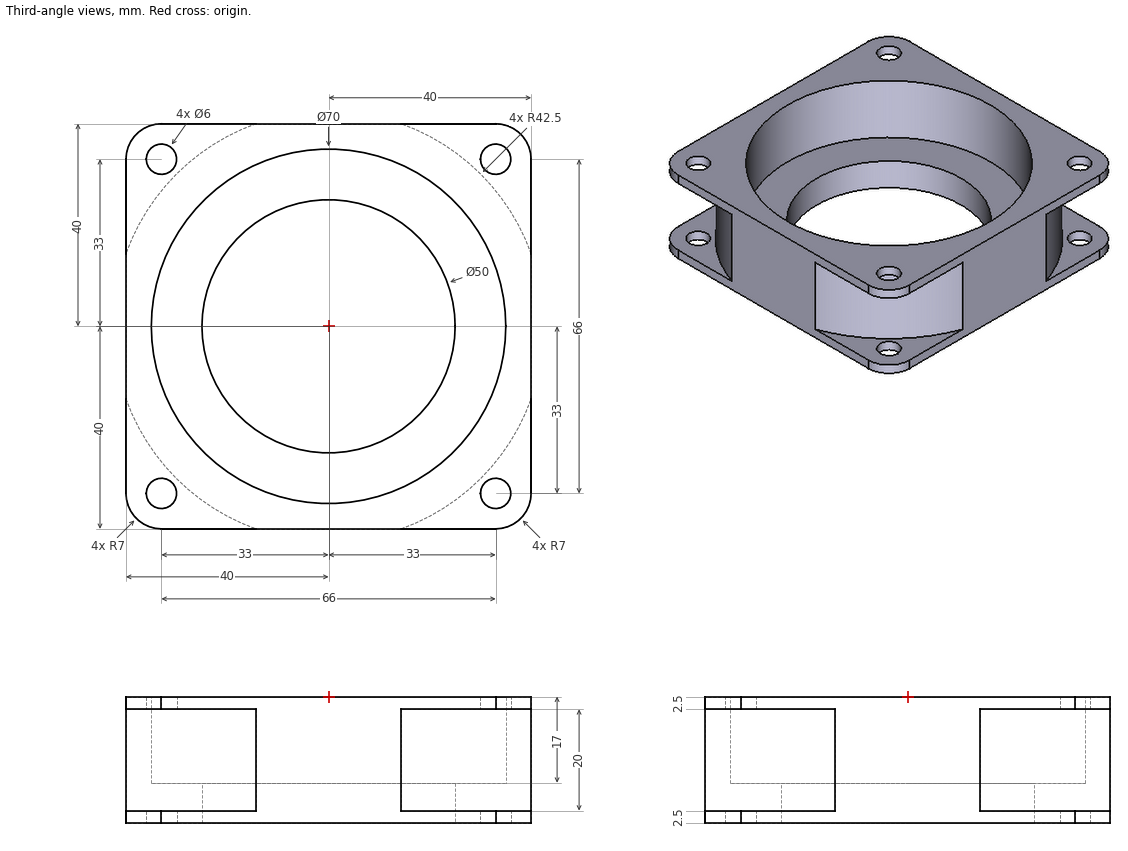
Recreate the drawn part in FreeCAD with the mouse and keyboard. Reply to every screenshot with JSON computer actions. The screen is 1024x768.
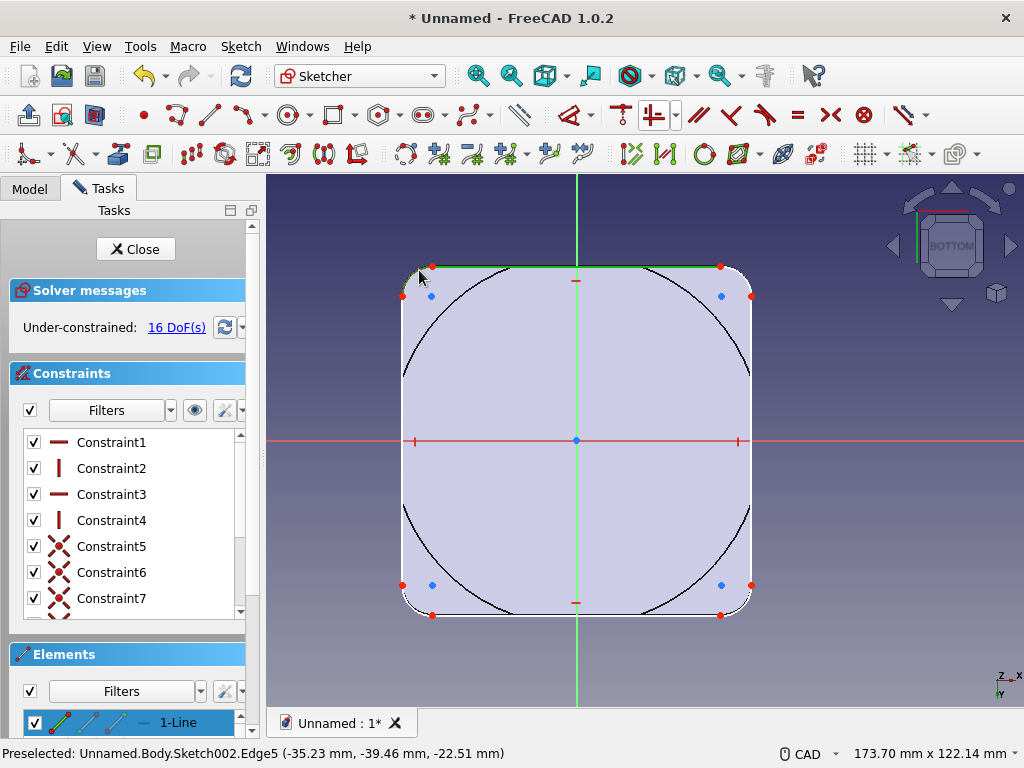
{"action": "left_click", "coordinate": [765, 116]}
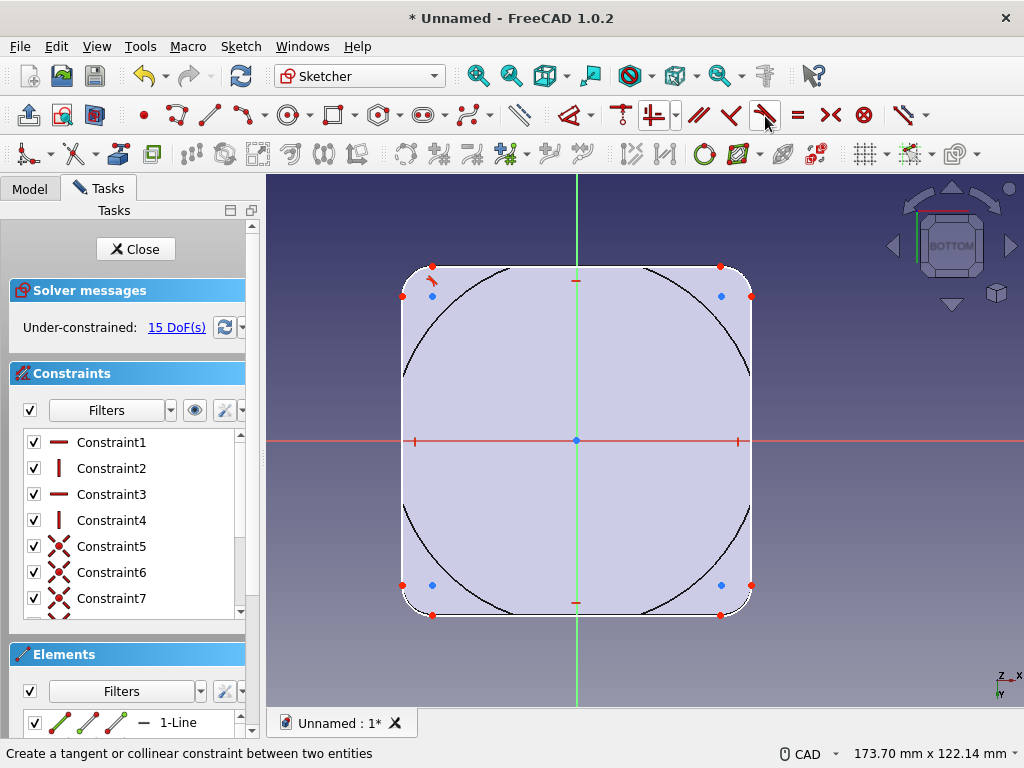
{"action": "left_click", "coordinate": [634, 267]}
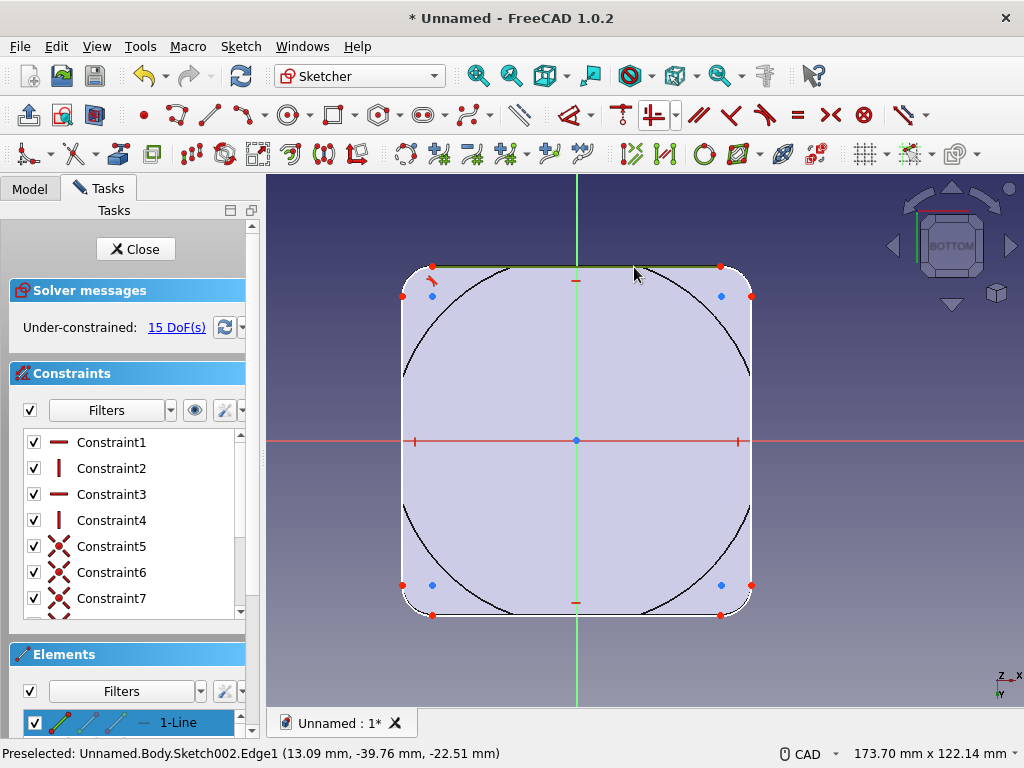
{"action": "left_click", "coordinate": [748, 283]}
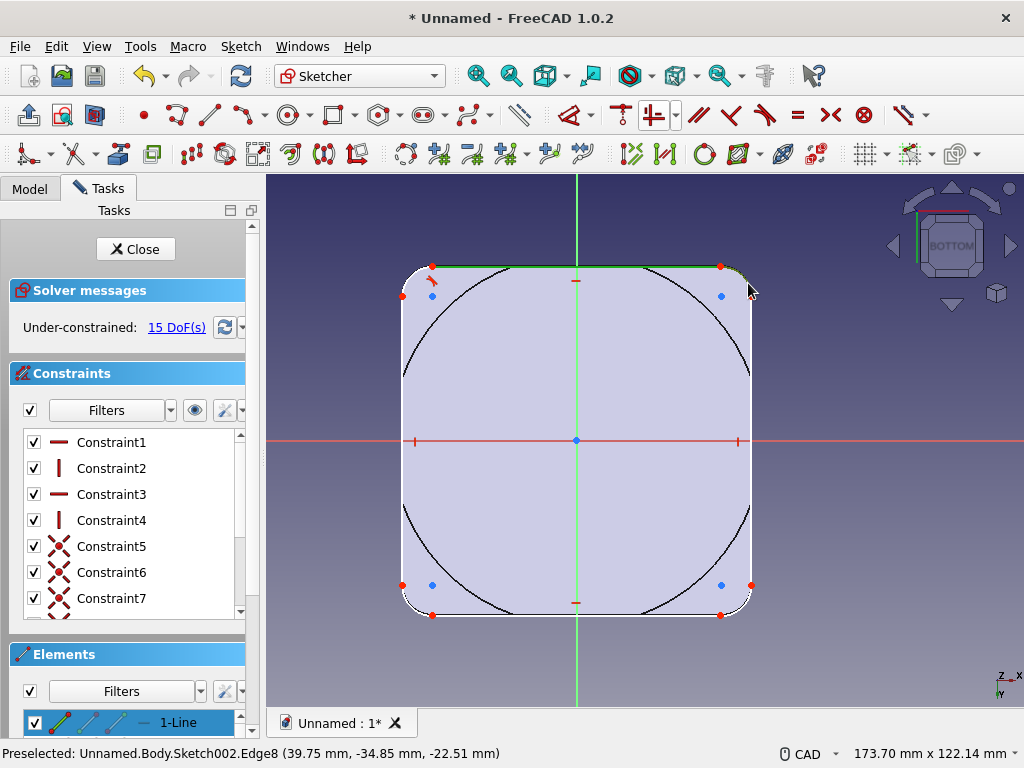
{"action": "left_click", "coordinate": [765, 116]}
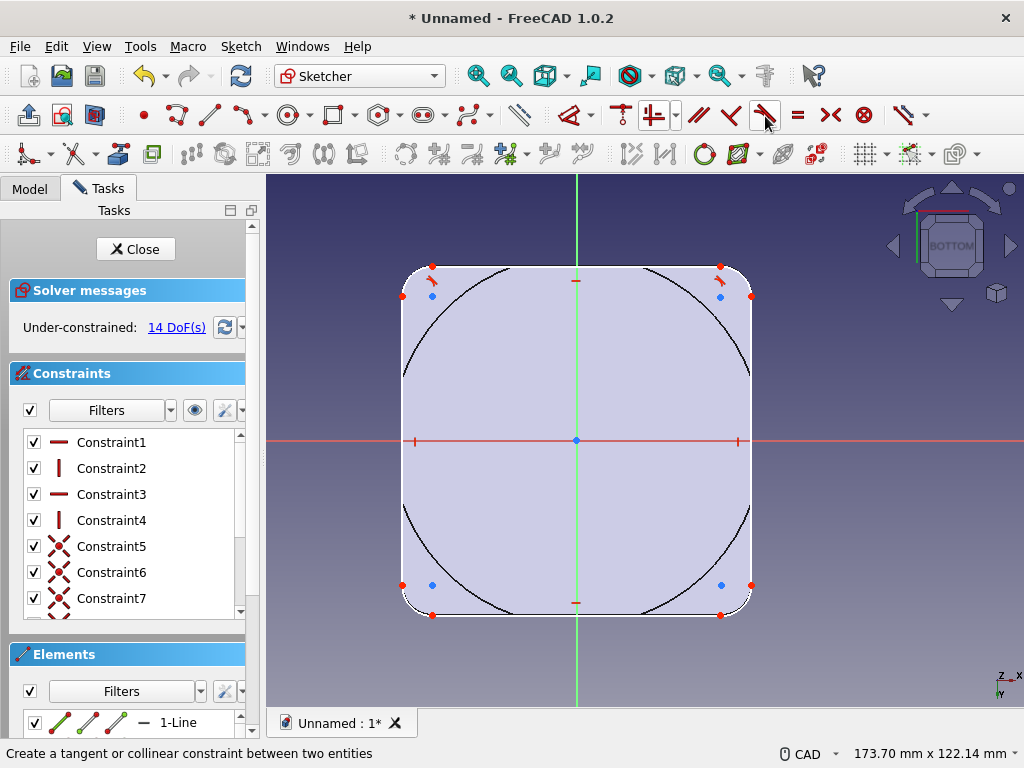
{"action": "left_click", "coordinate": [402, 384]}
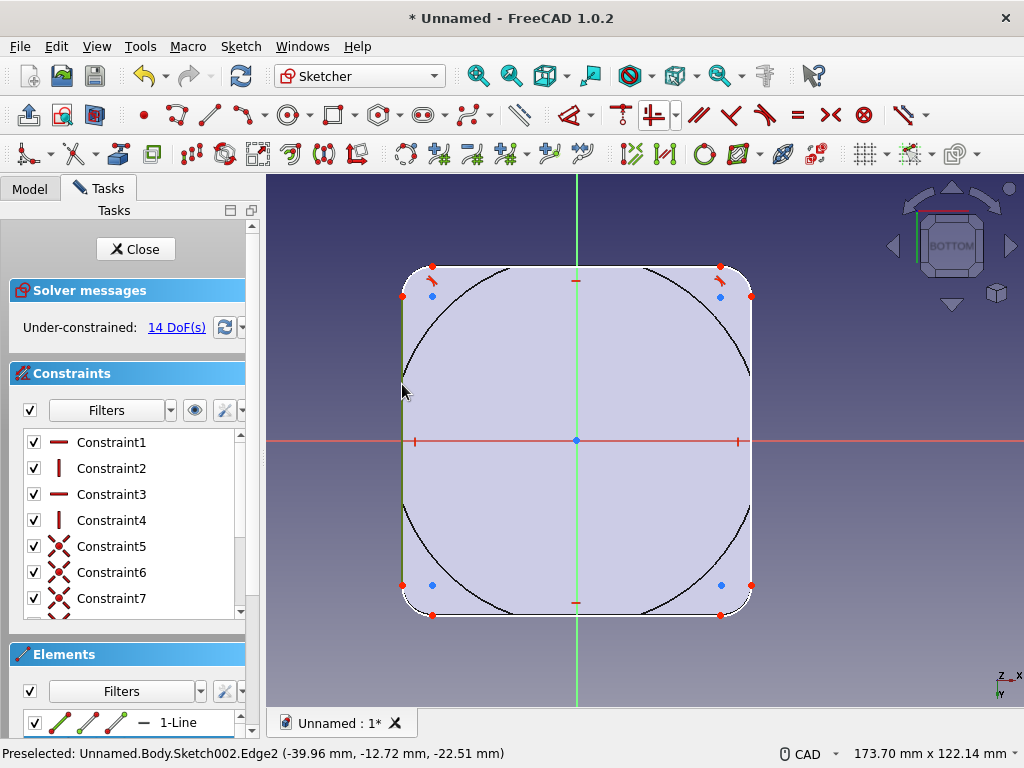
{"action": "left_click", "coordinate": [419, 270]}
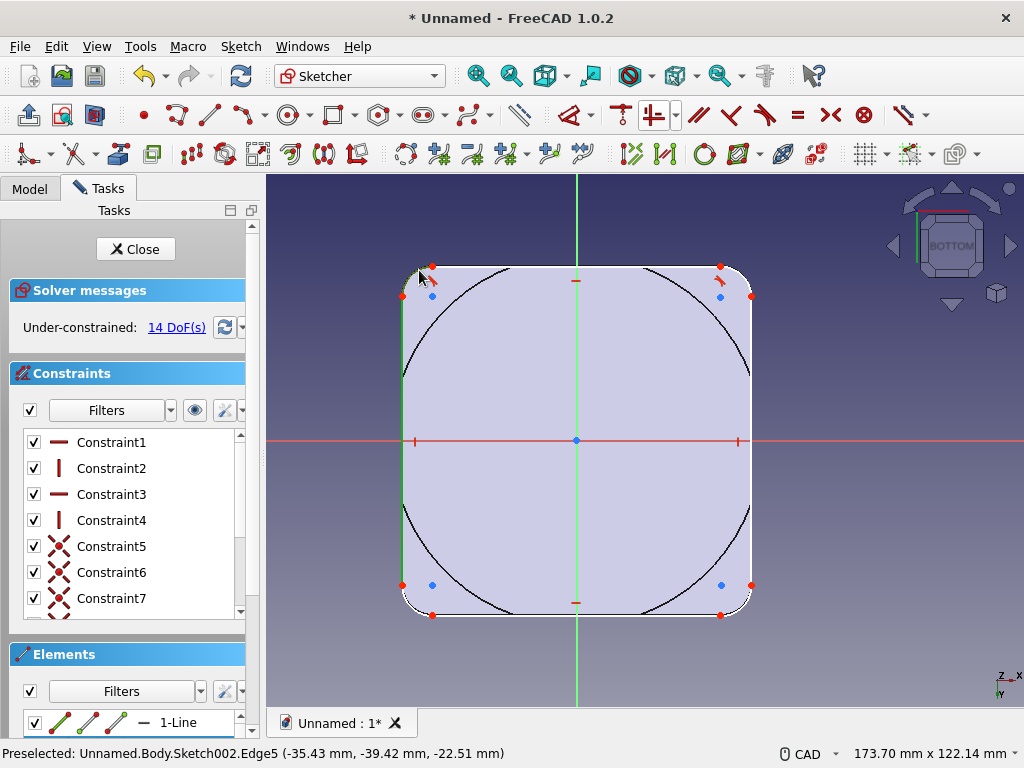
{"action": "left_click", "coordinate": [765, 116]}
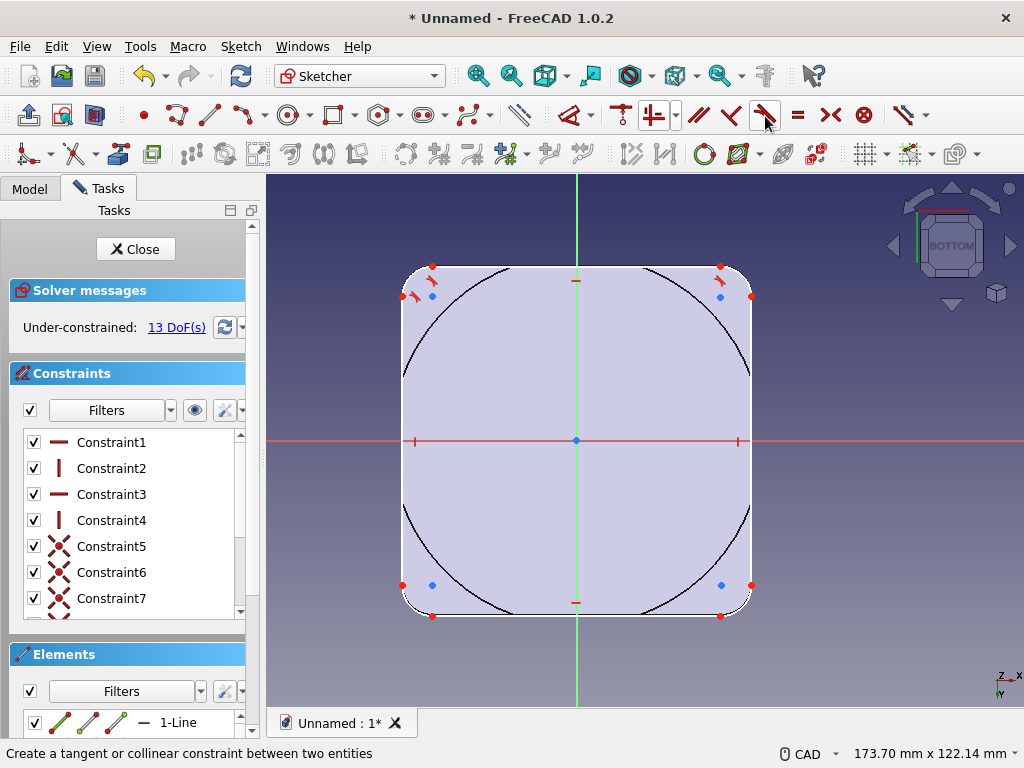
{"action": "left_click", "coordinate": [402, 384]}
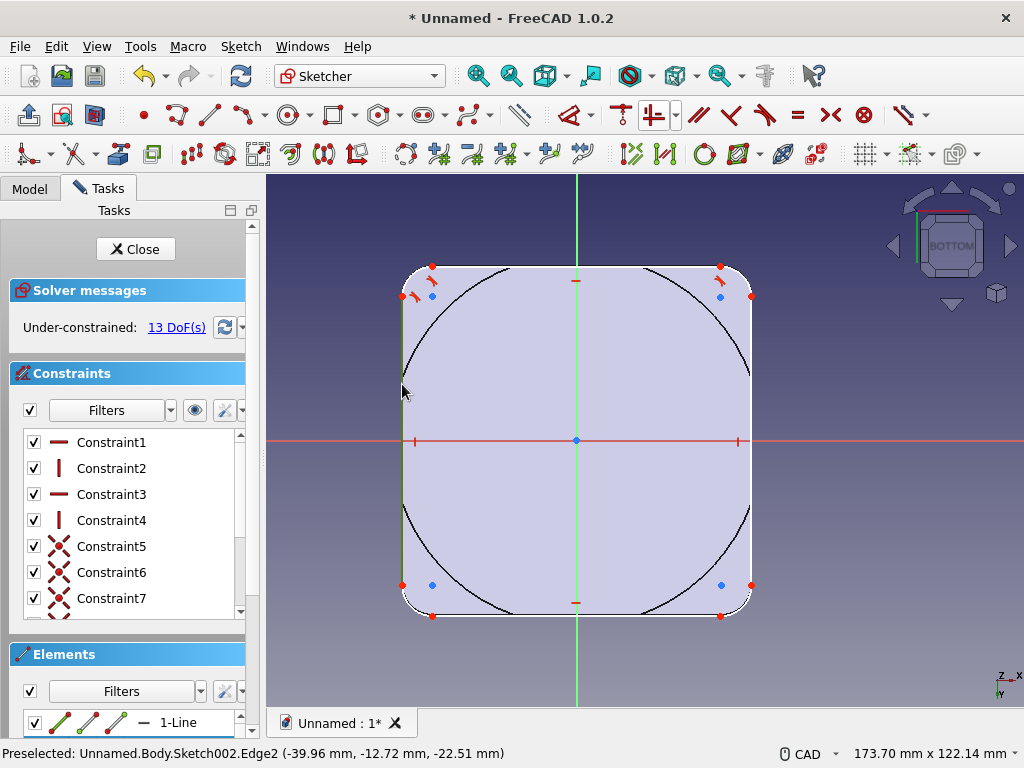
{"action": "left_click", "coordinate": [406, 600]}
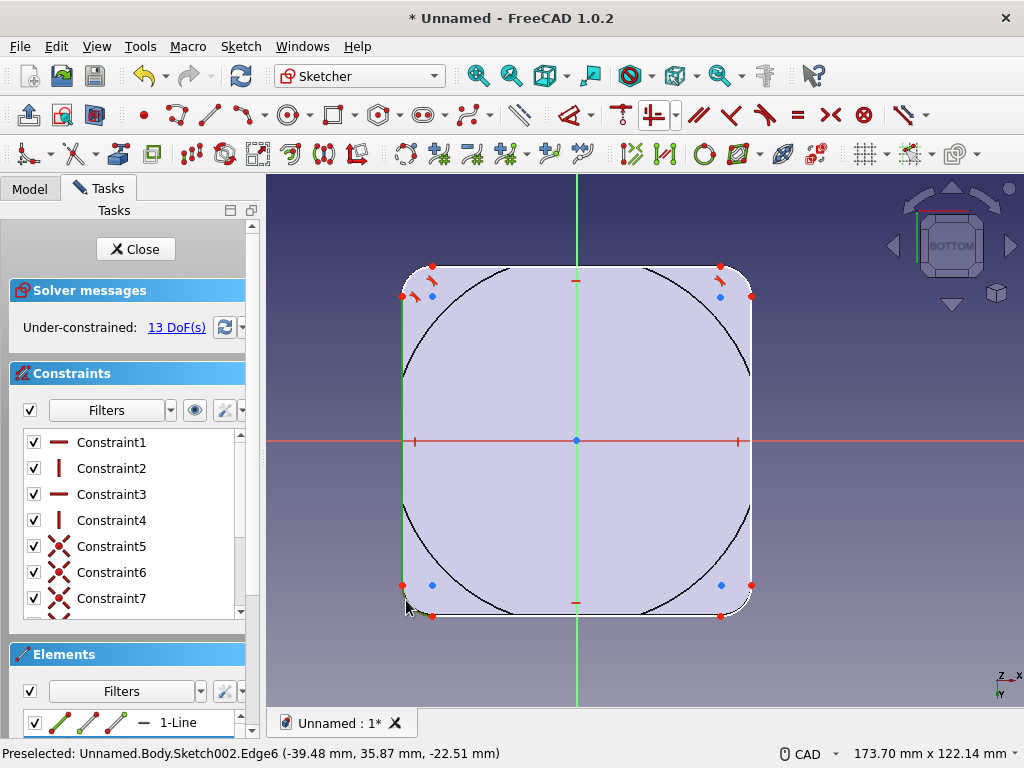
{"action": "left_click", "coordinate": [765, 116]}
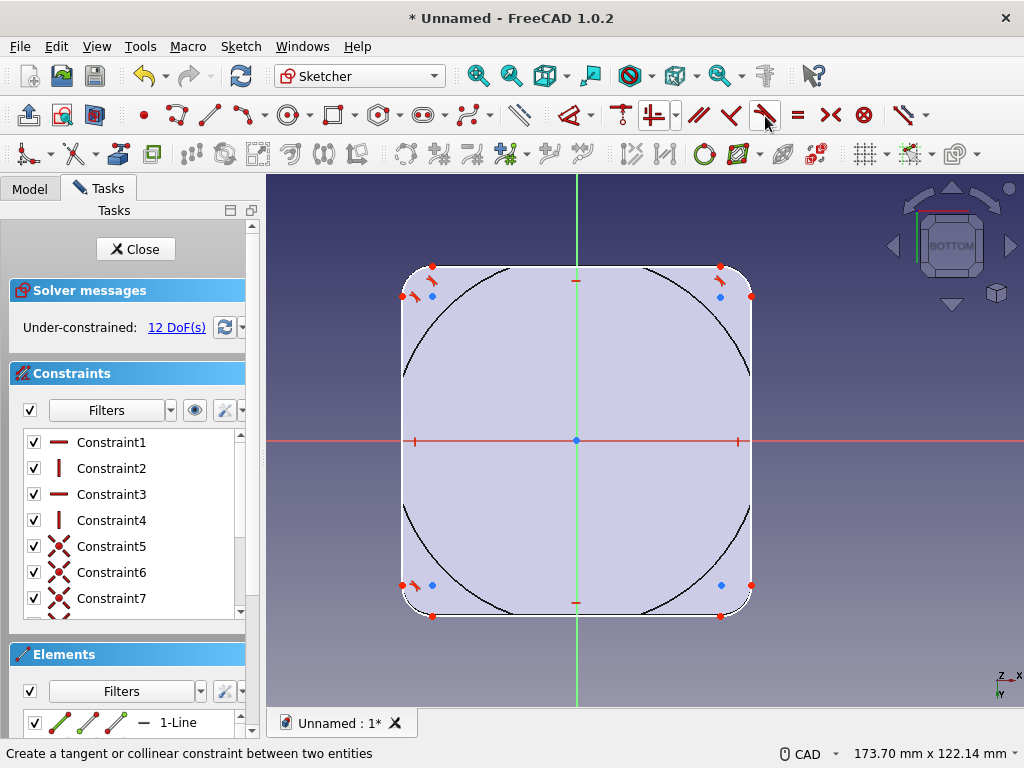
{"action": "left_click", "coordinate": [519, 616]}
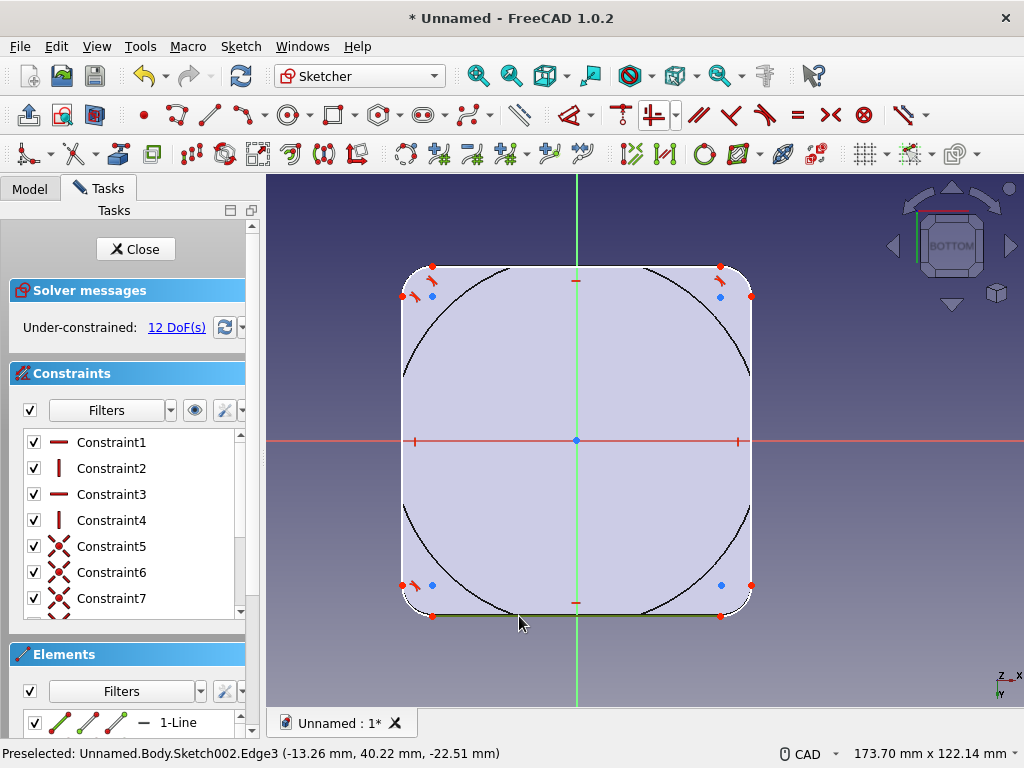
{"action": "left_click", "coordinate": [406, 600]}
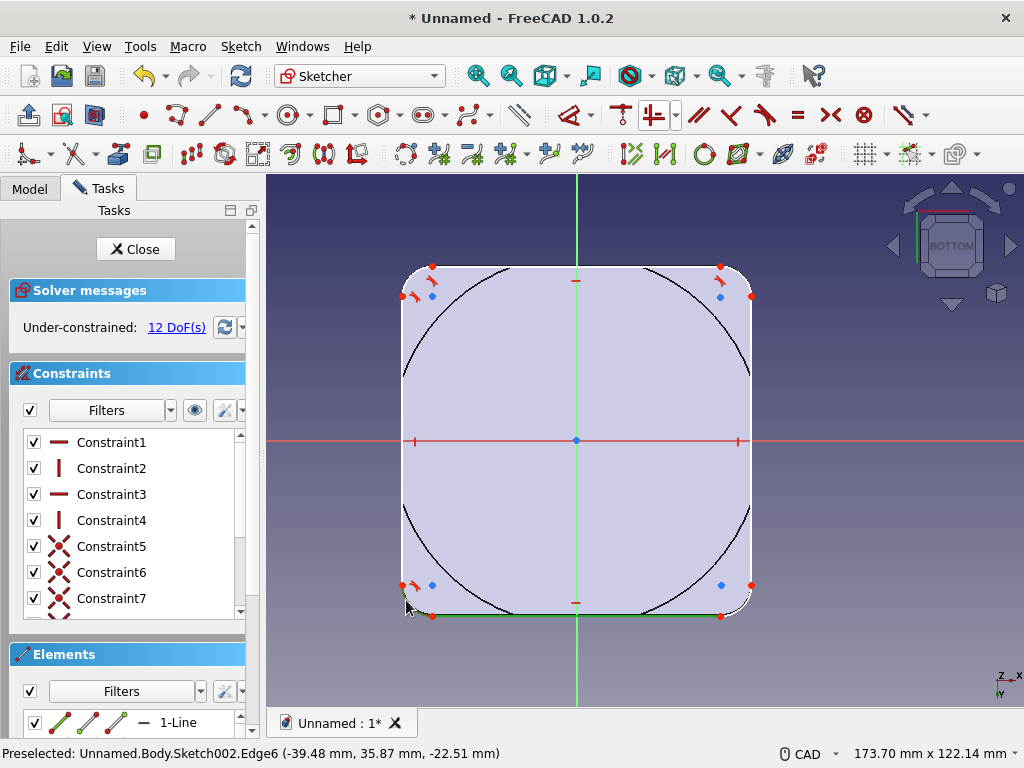
{"action": "left_click", "coordinate": [765, 116]}